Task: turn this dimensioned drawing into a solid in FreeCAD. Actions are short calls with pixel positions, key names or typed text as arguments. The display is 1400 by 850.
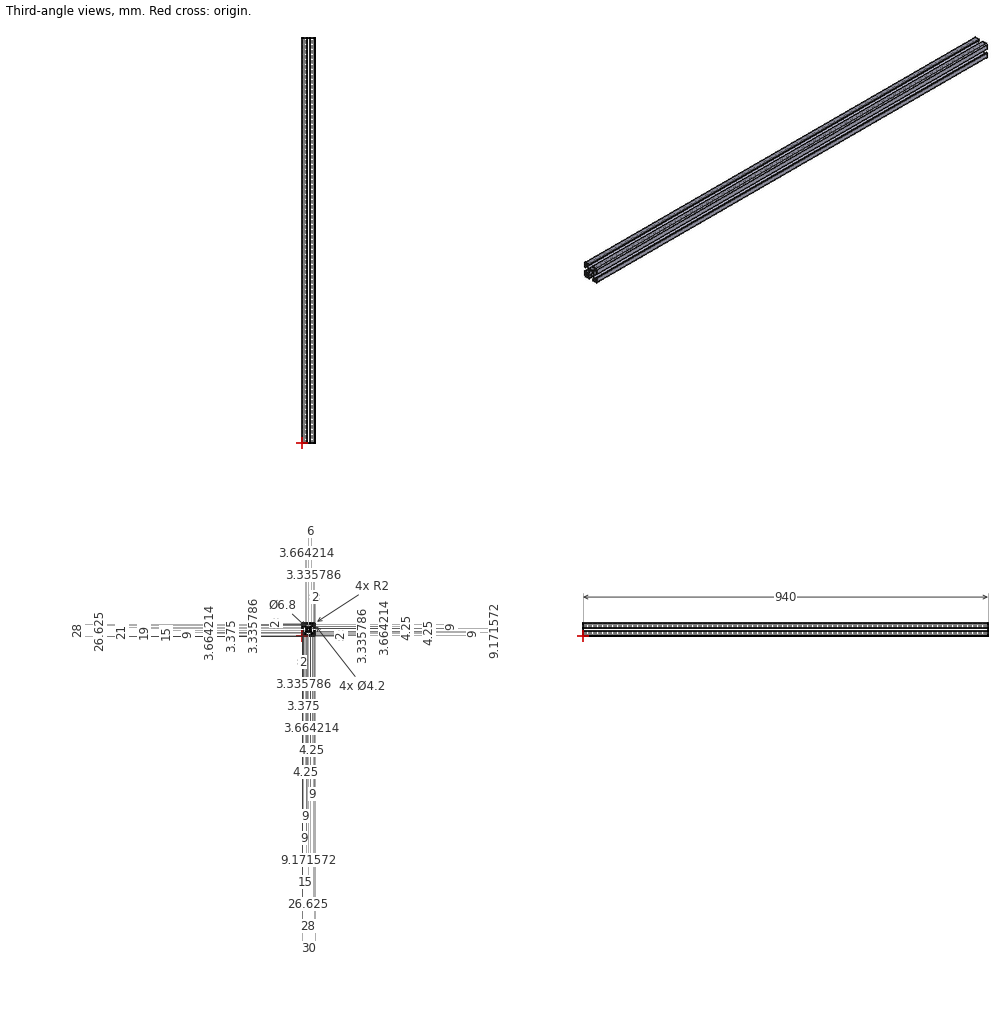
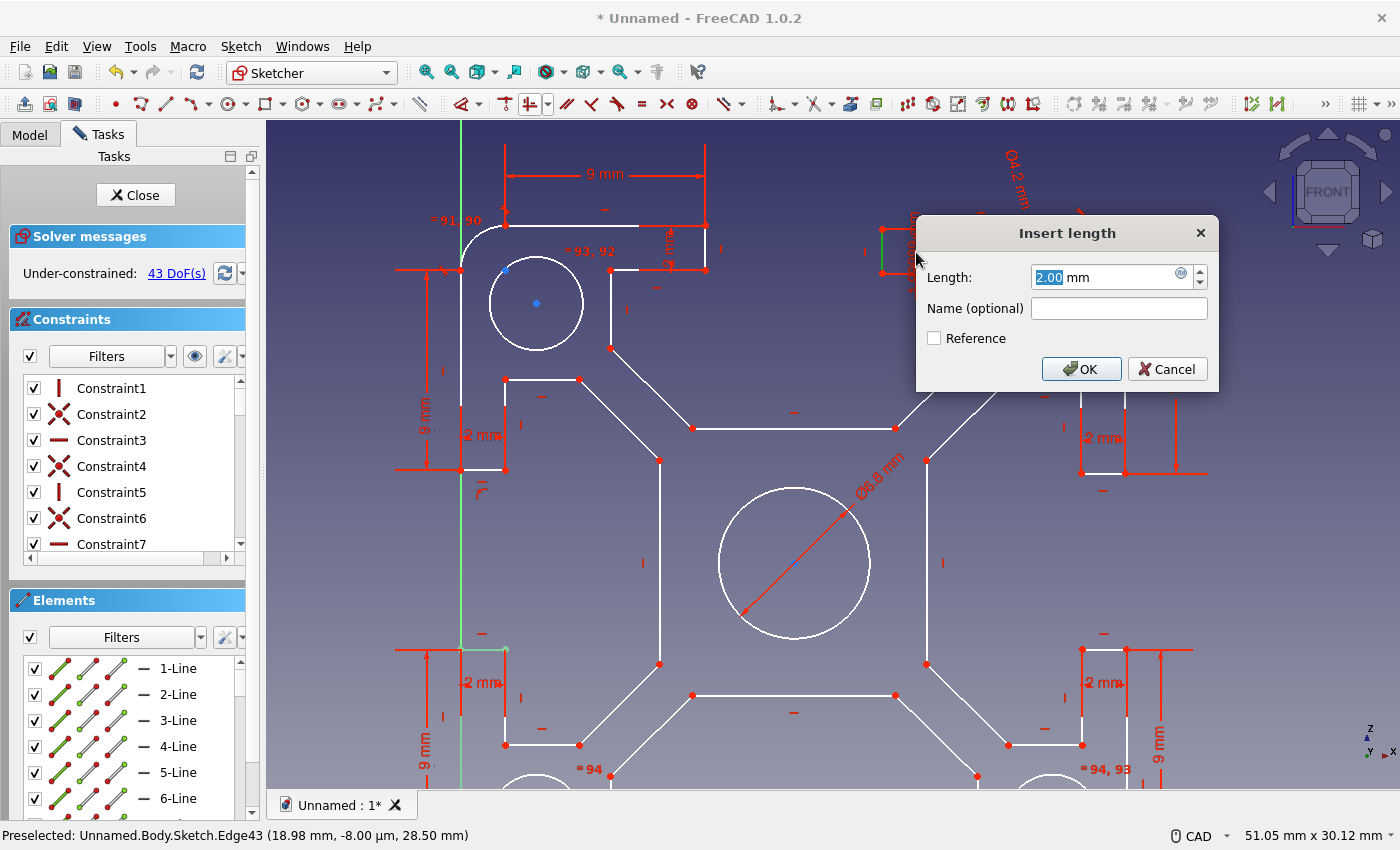
text(2)
key(Return)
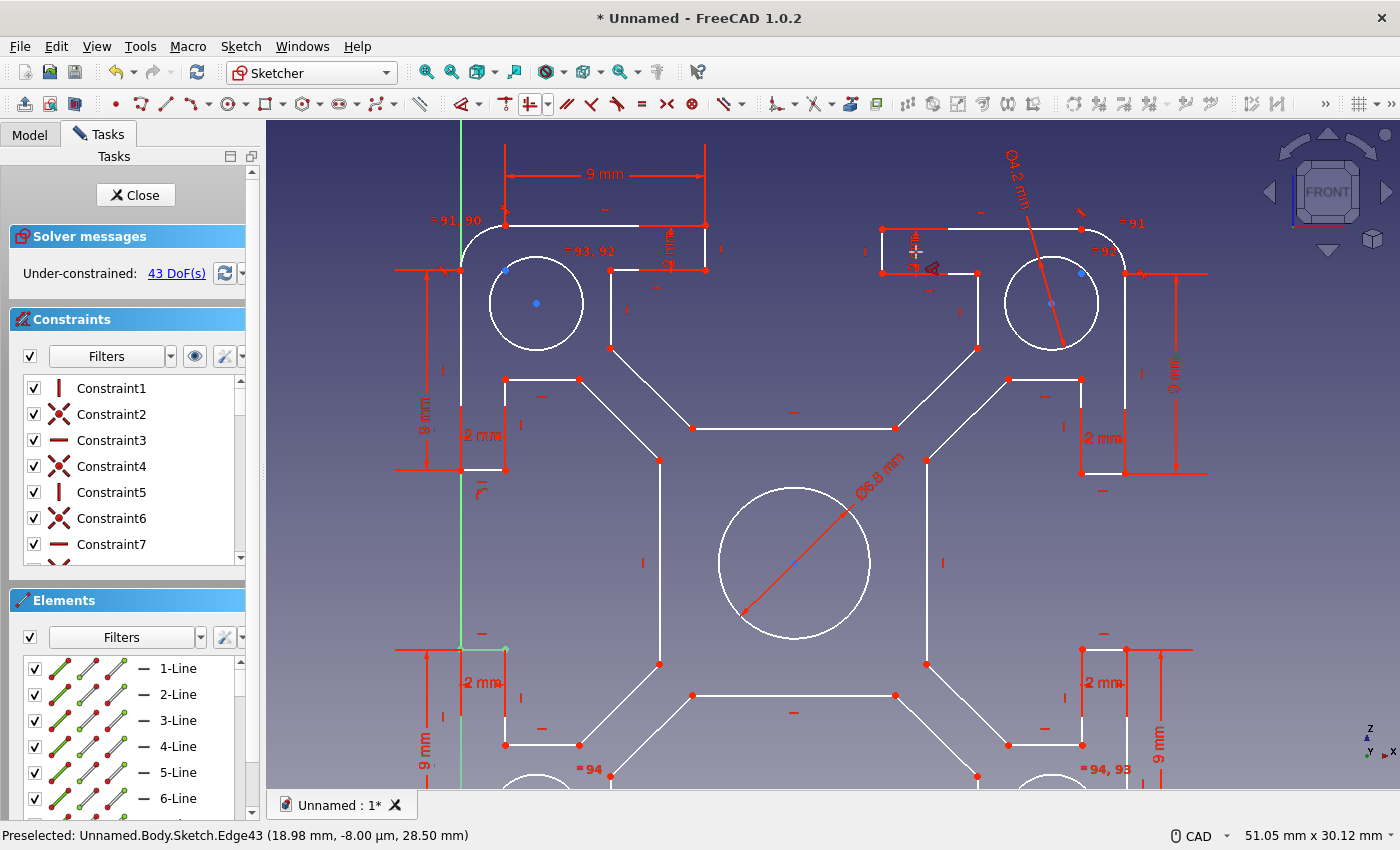
click(942, 229)
click(936, 195)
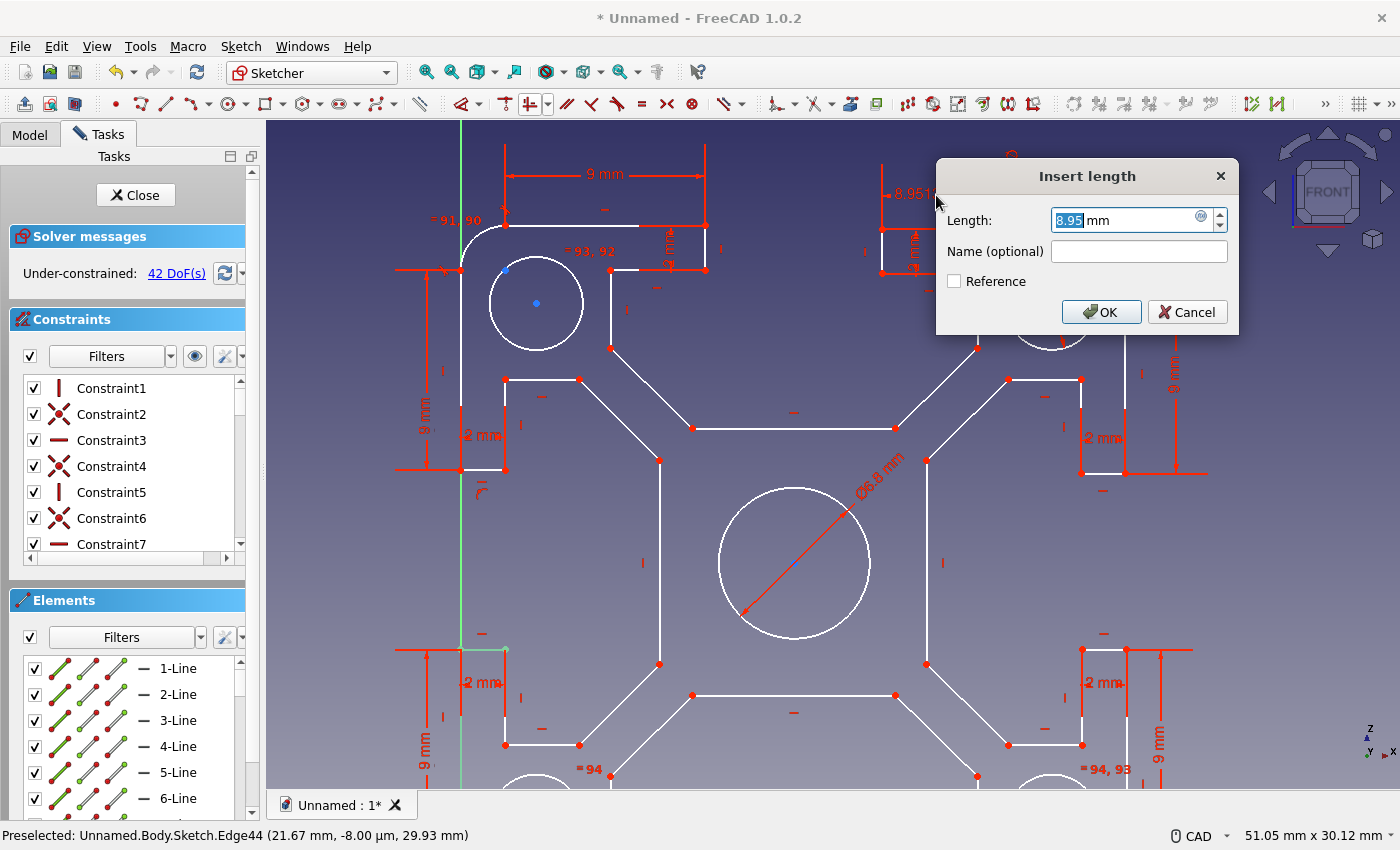
text(9)
key(Return)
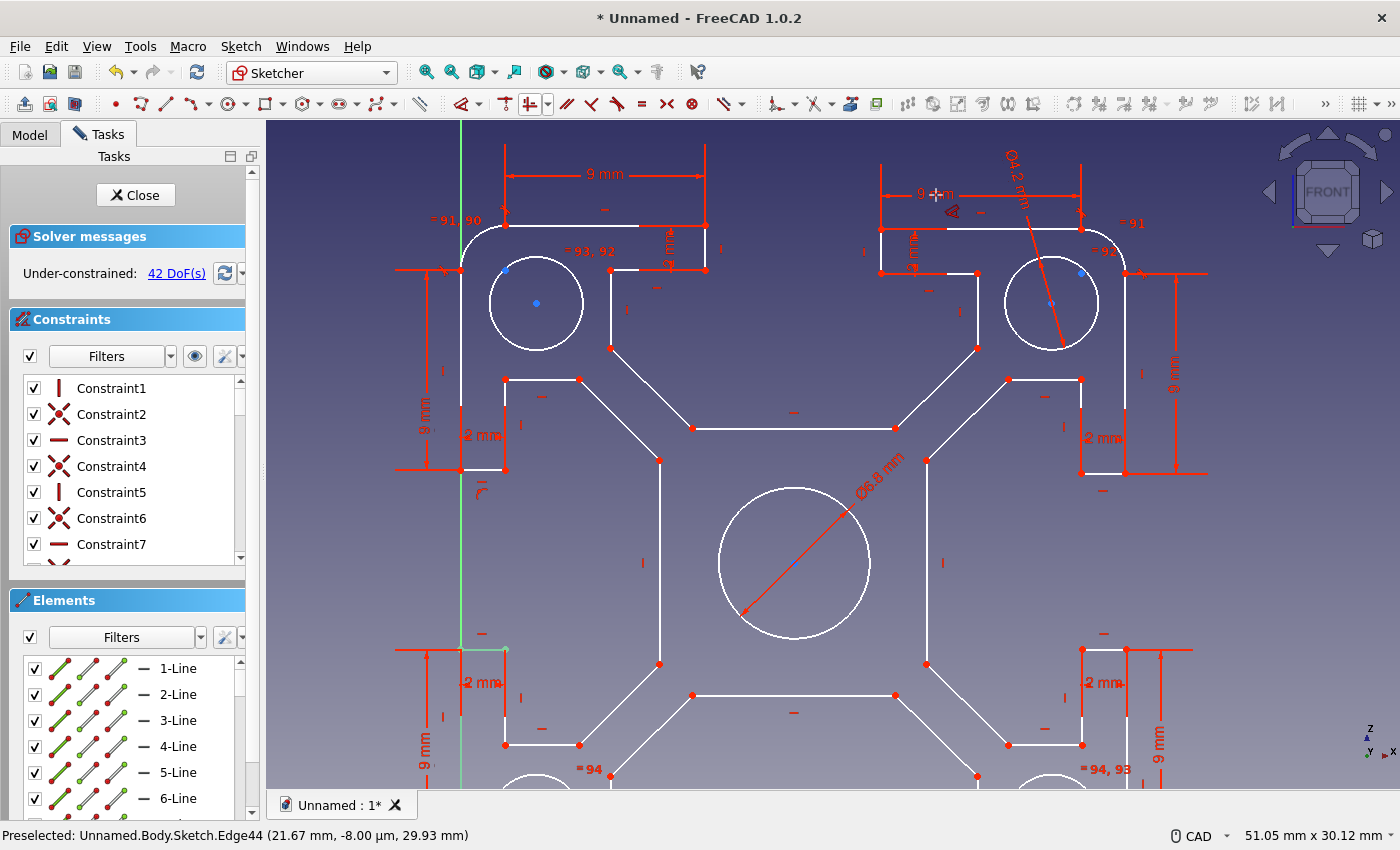
click(896, 696)
click(427, 728)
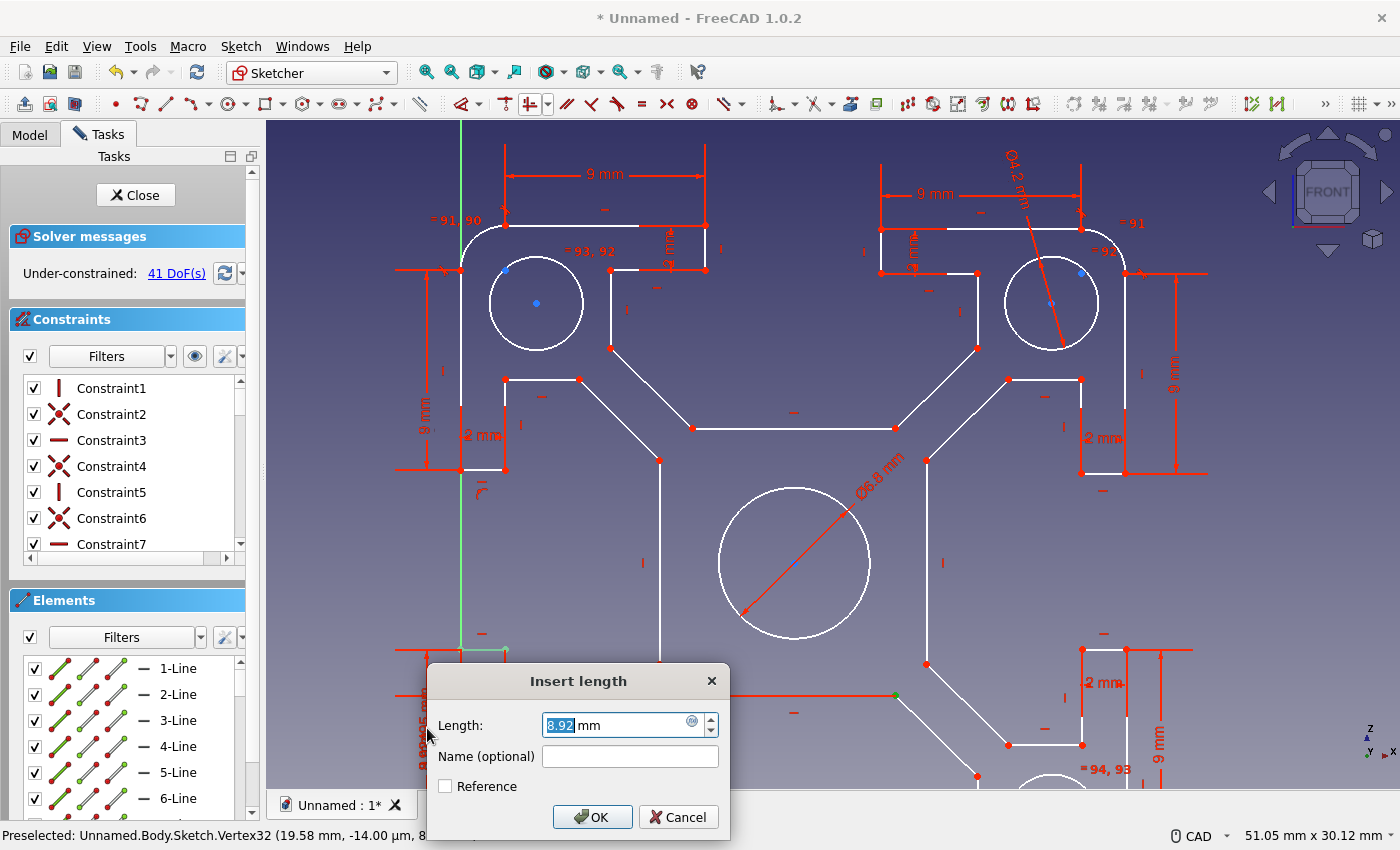
text(9)
key(Return)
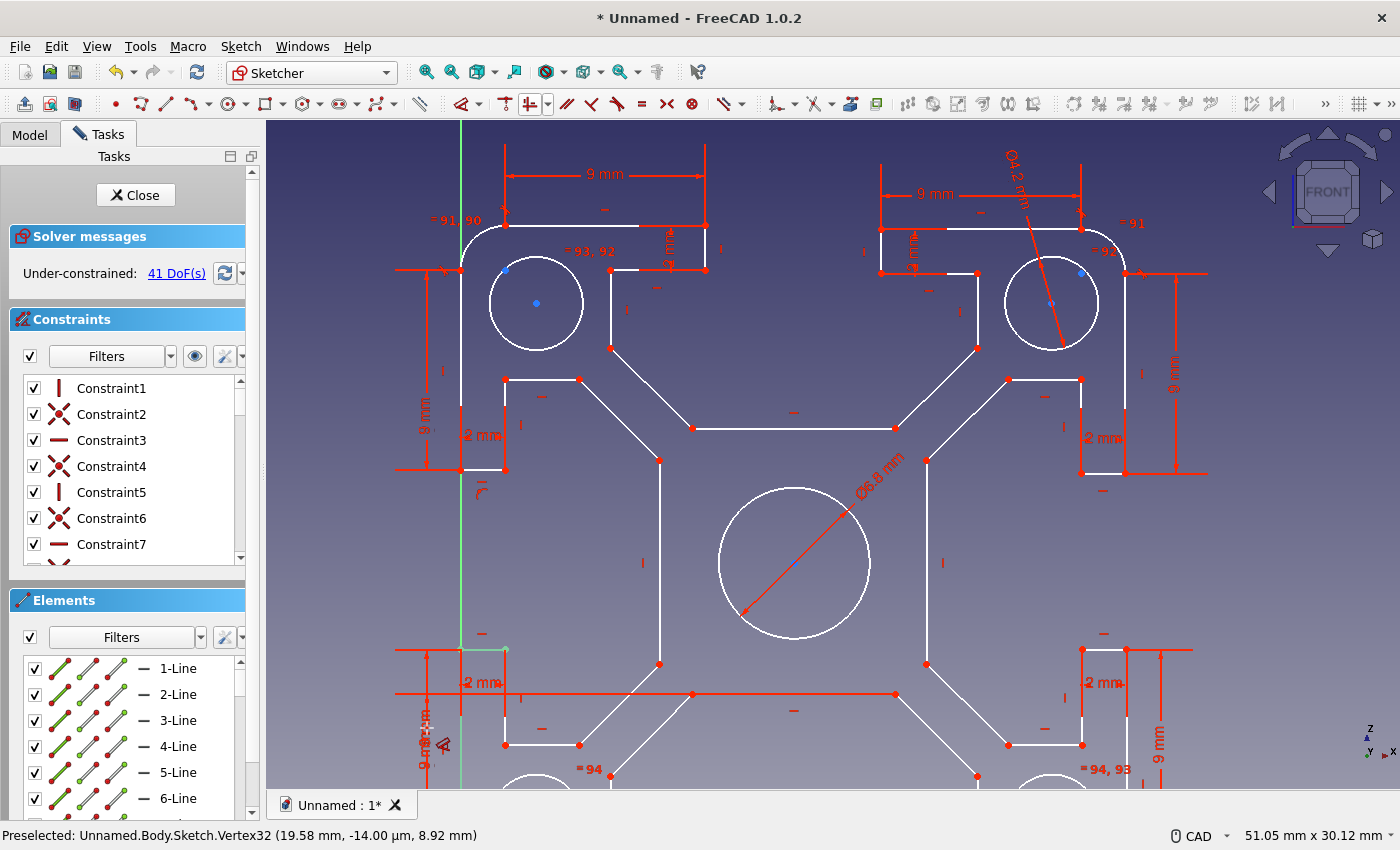
click(660, 665)
click(560, 631)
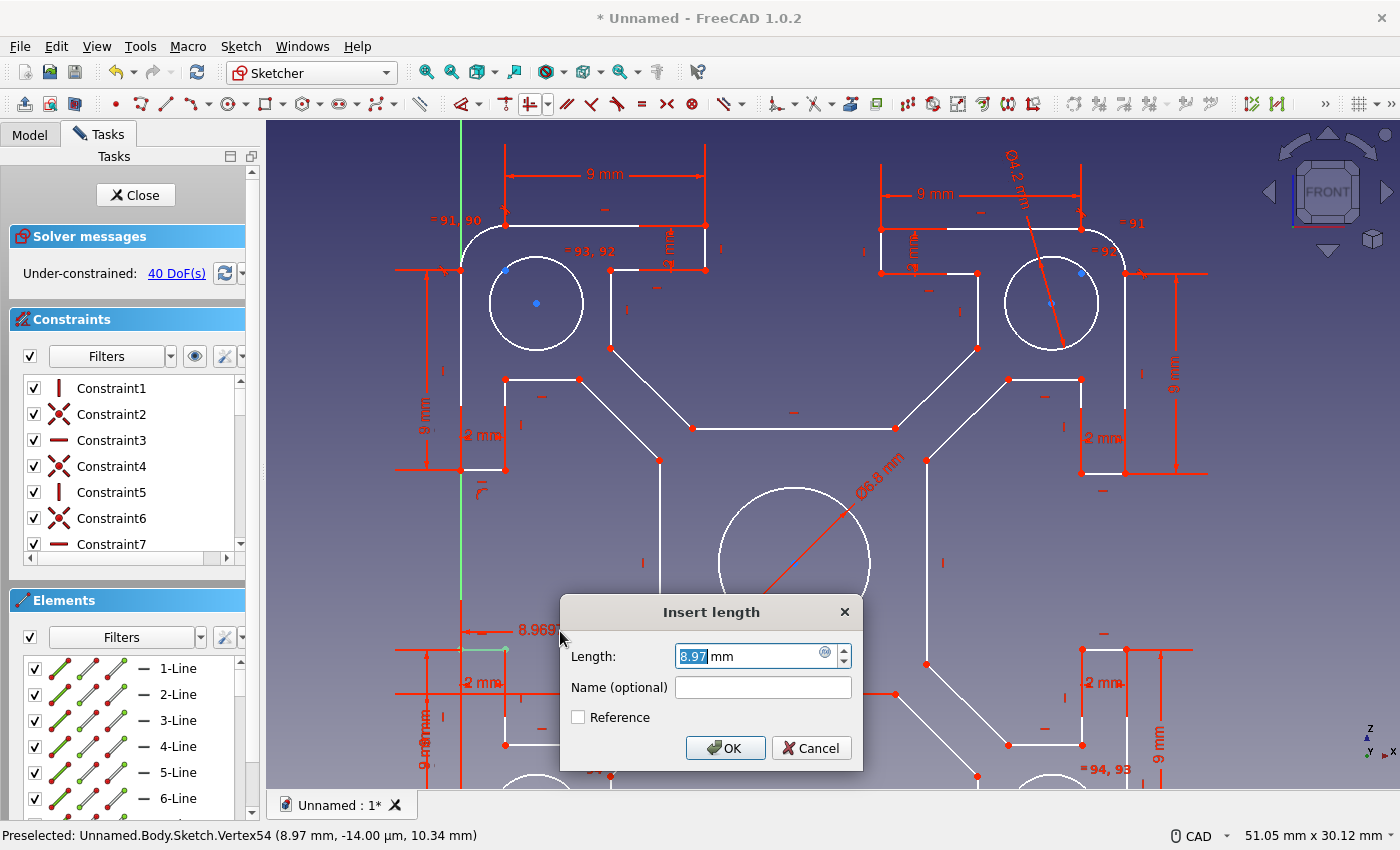
text(9)
key(Return)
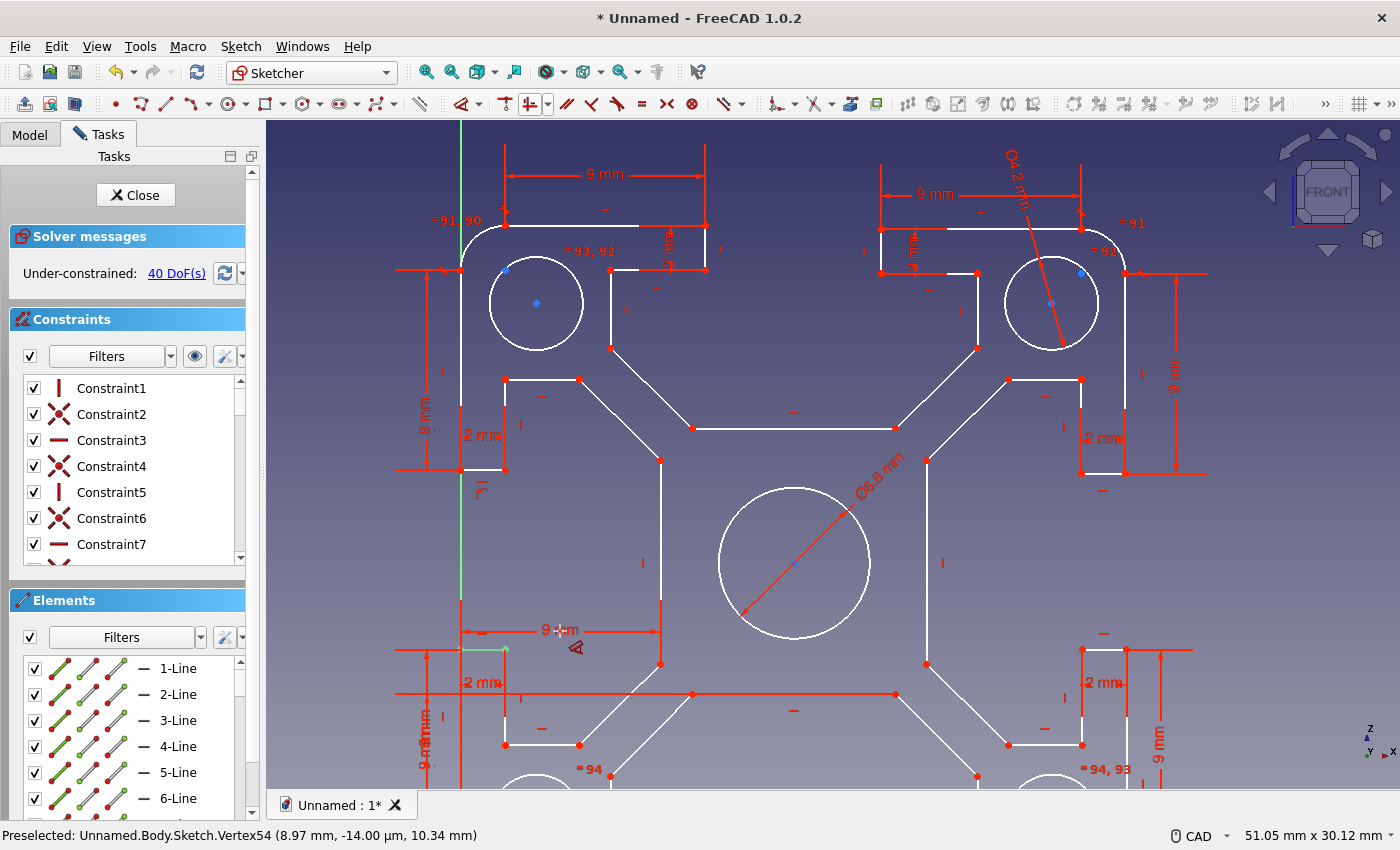
click(794, 563)
click(627, 529)